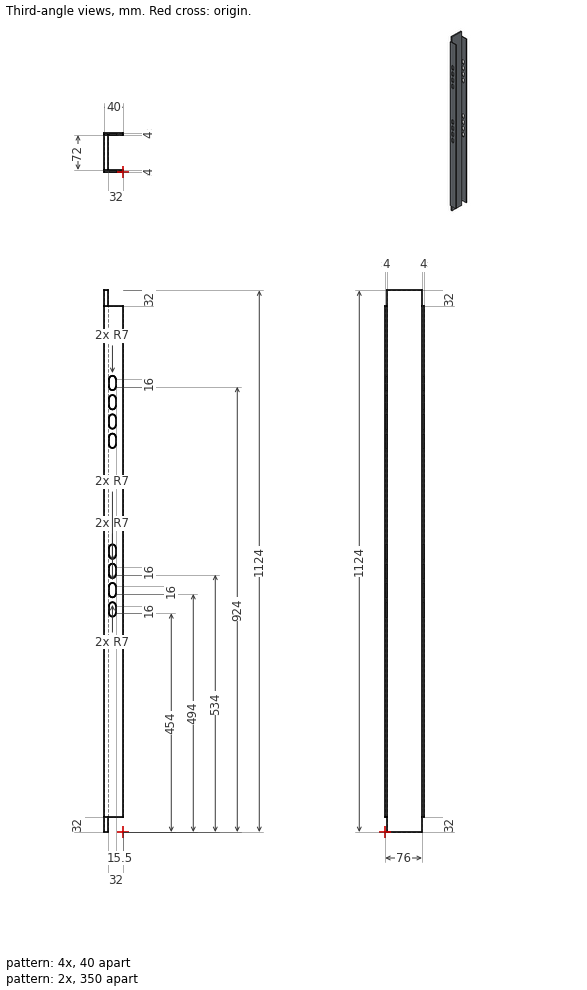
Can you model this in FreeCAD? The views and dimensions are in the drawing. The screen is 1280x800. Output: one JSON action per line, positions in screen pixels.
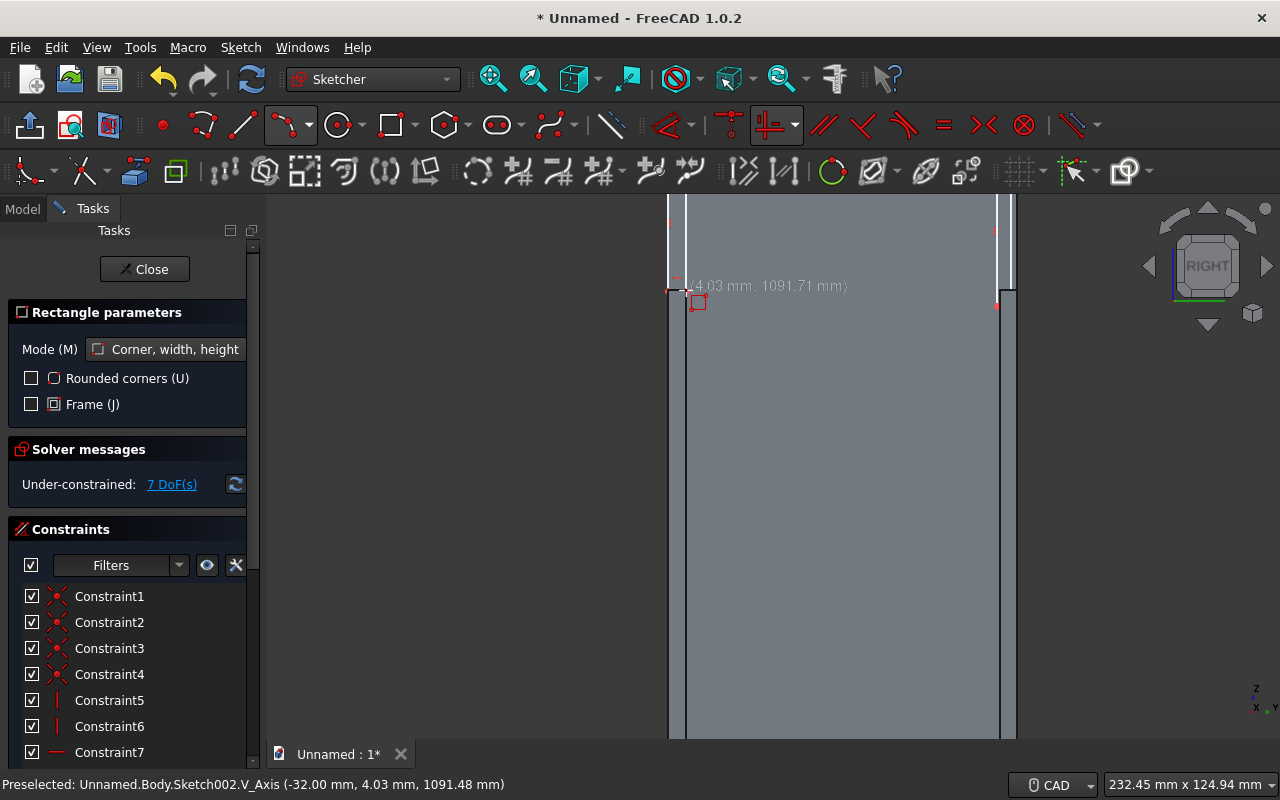
{"action": "scroll", "coordinate": [693, 295], "scroll_direction": "down", "scroll_amount": 13}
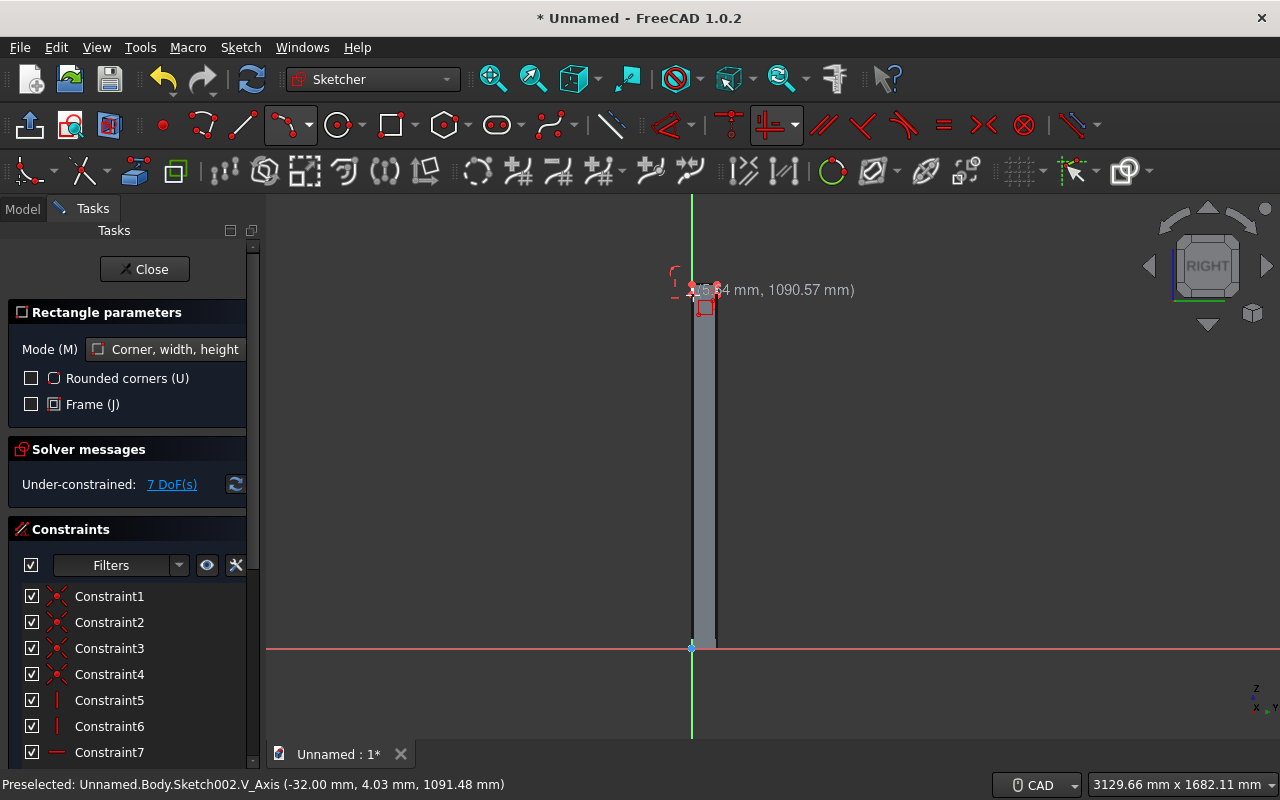
{"action": "scroll", "coordinate": [716, 638], "scroll_direction": "up", "scroll_amount": 13}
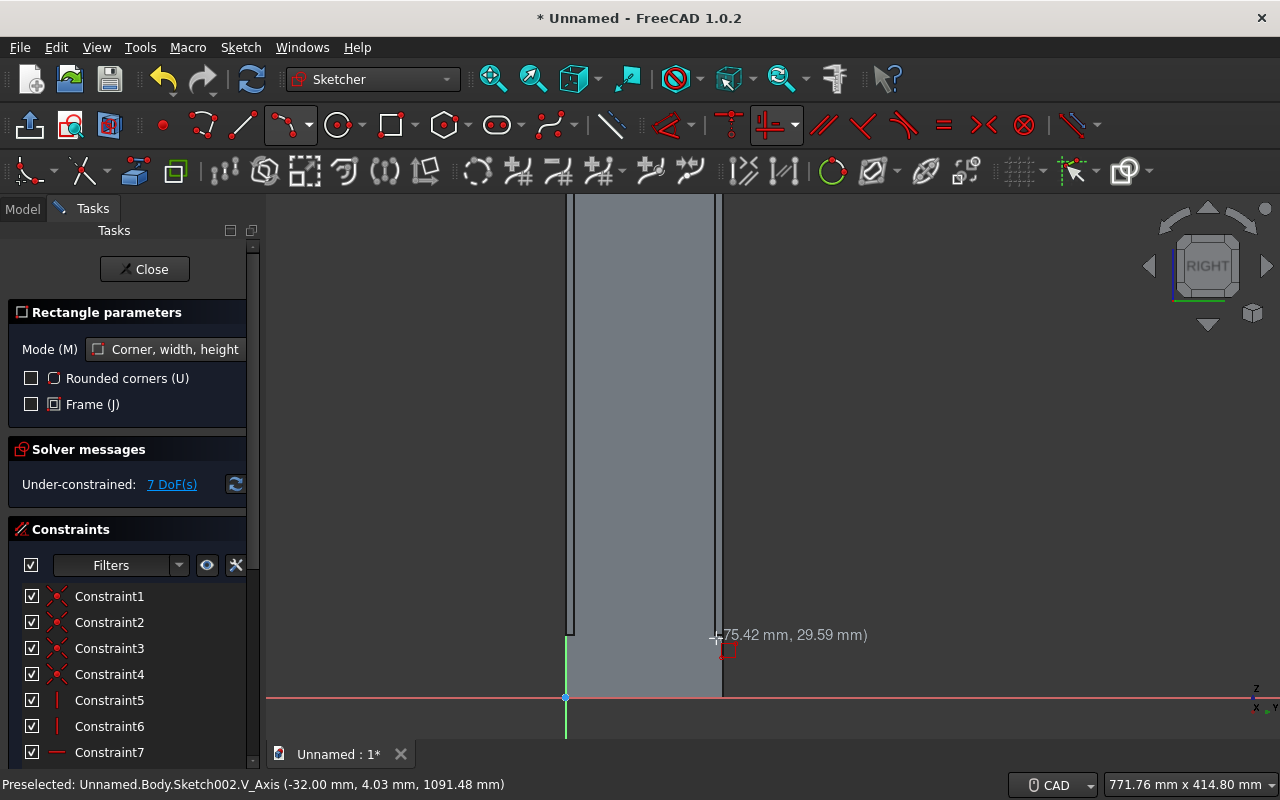
{"action": "scroll", "coordinate": [716, 639], "scroll_direction": "down", "scroll_amount": 13}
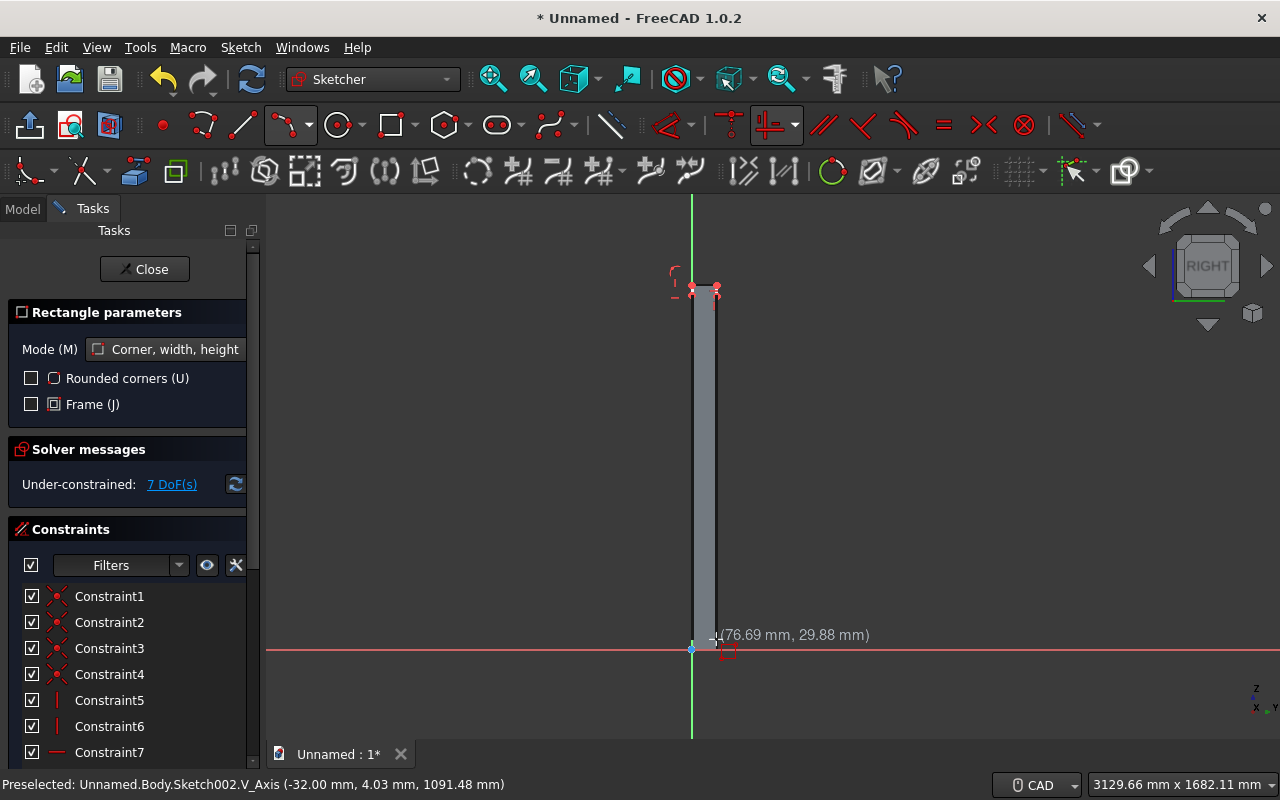
{"action": "scroll", "coordinate": [716, 639], "scroll_direction": "up", "scroll_amount": 3}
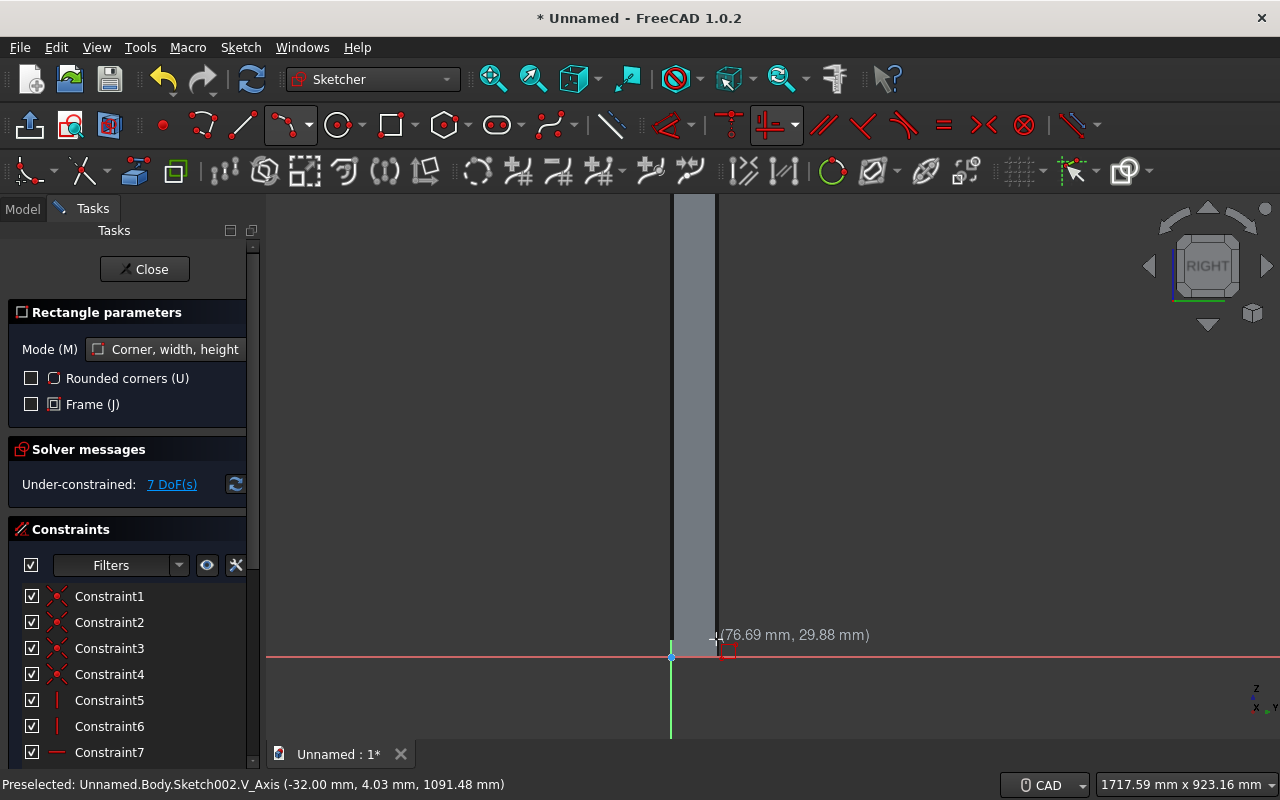
{"action": "left_click", "coordinate": [716, 639]}
{"action": "left_click", "coordinate": [718, 657]}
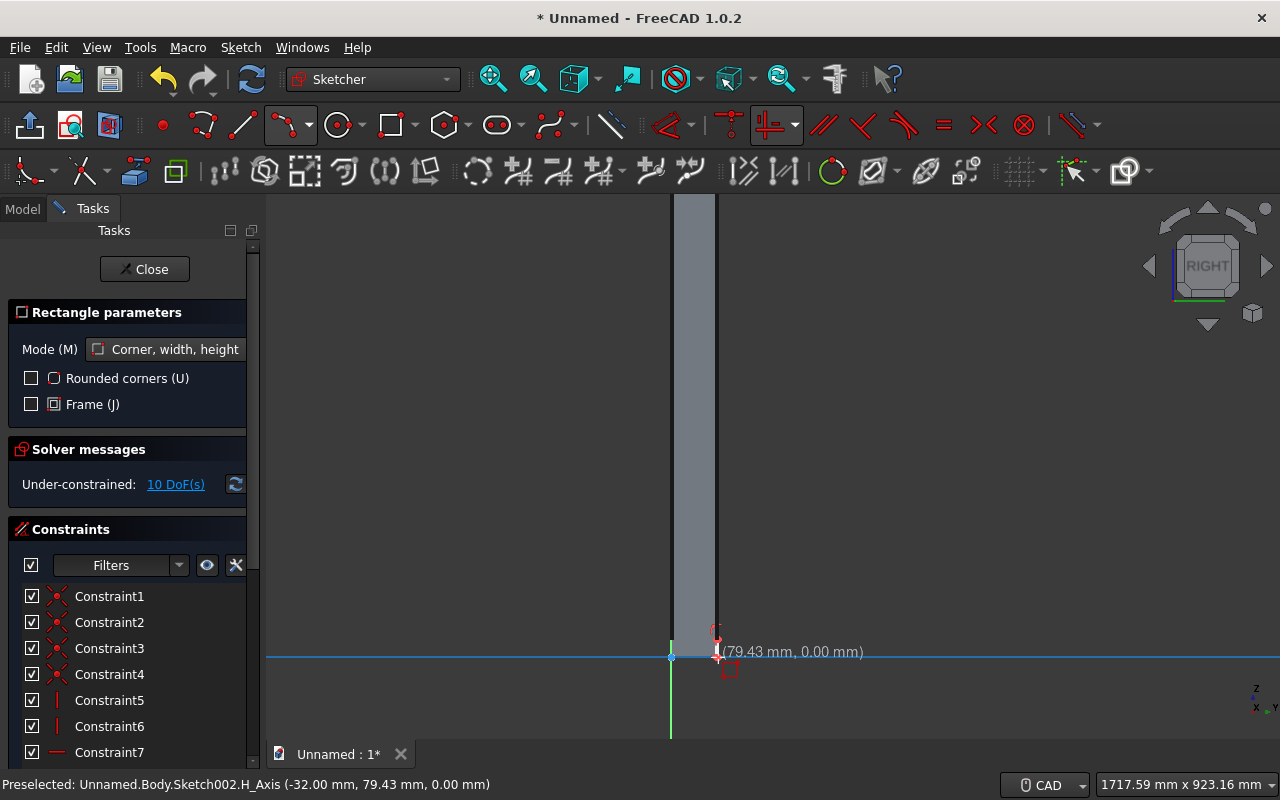
{"action": "scroll", "coordinate": [671, 657], "scroll_direction": "up", "scroll_amount": 10}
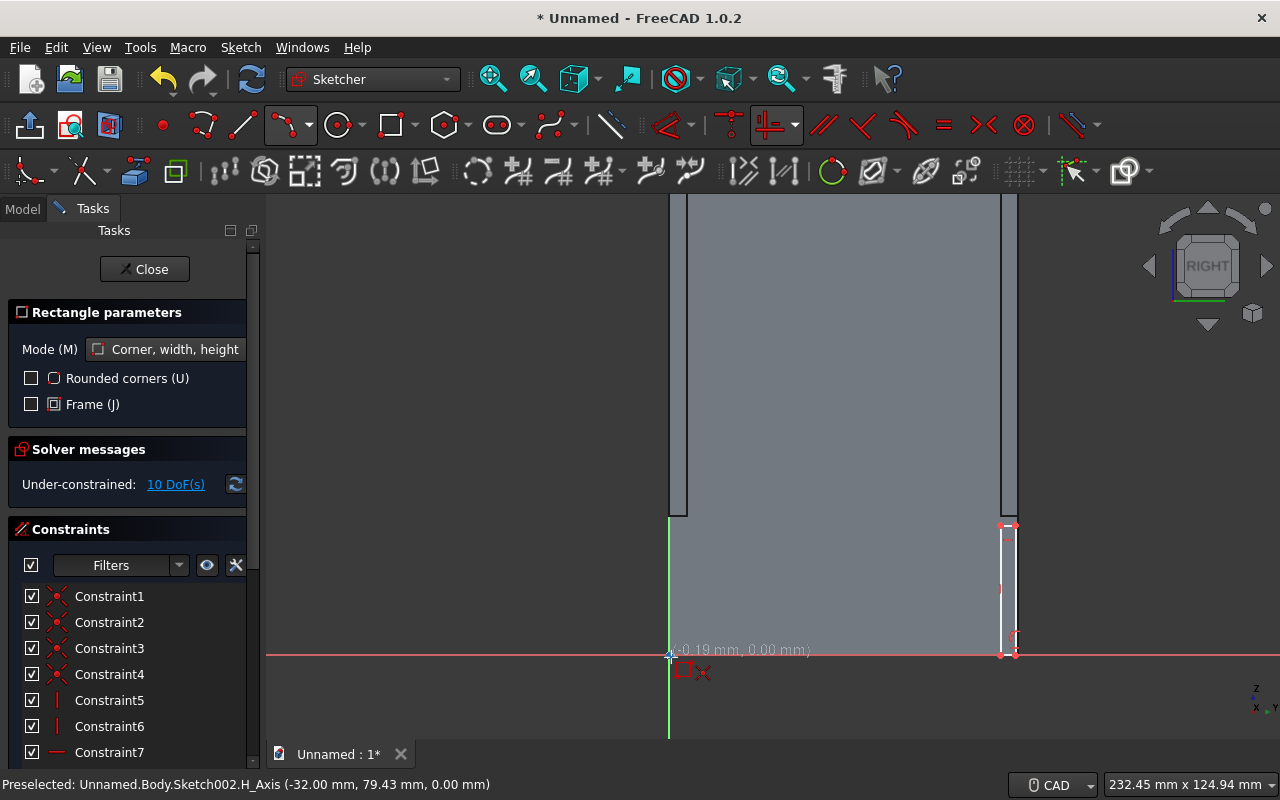
{"action": "scroll", "coordinate": [693, 648], "scroll_direction": "down", "scroll_amount": 13}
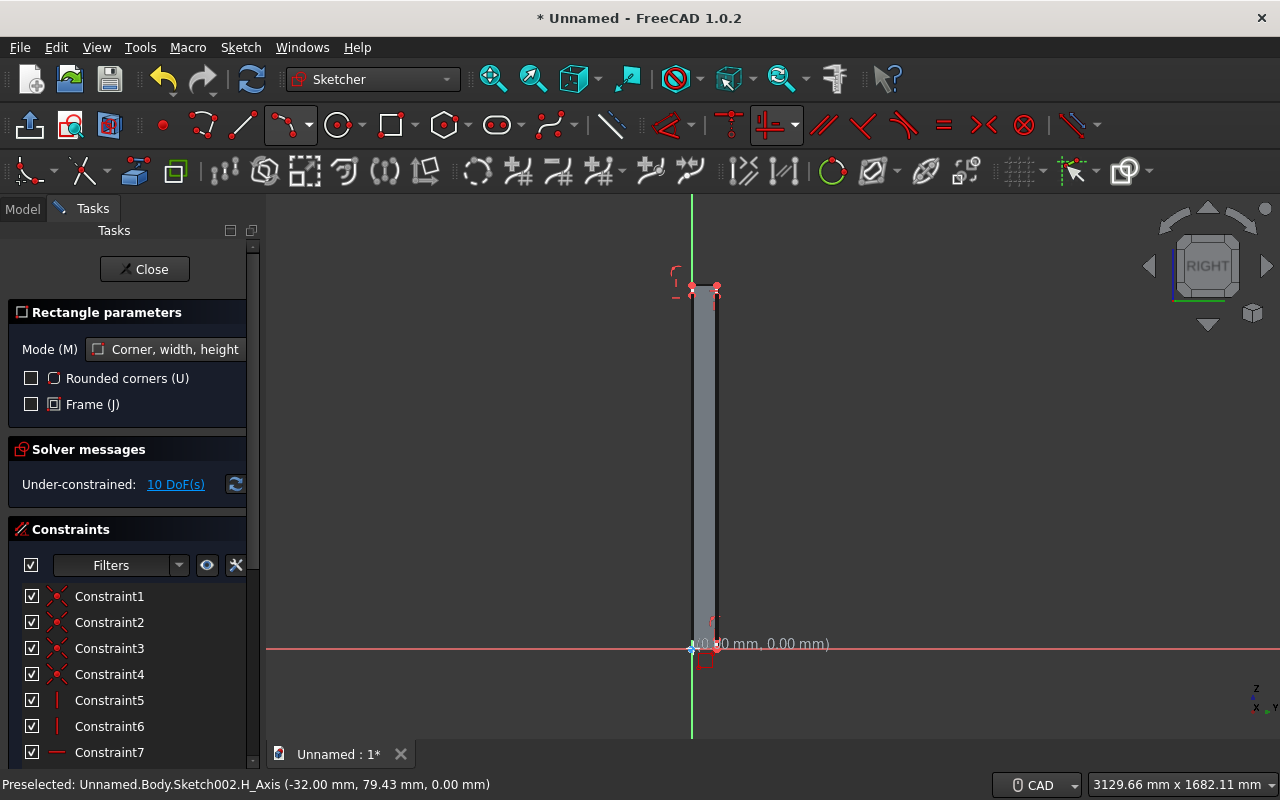
{"action": "left_click", "coordinate": [692, 649]}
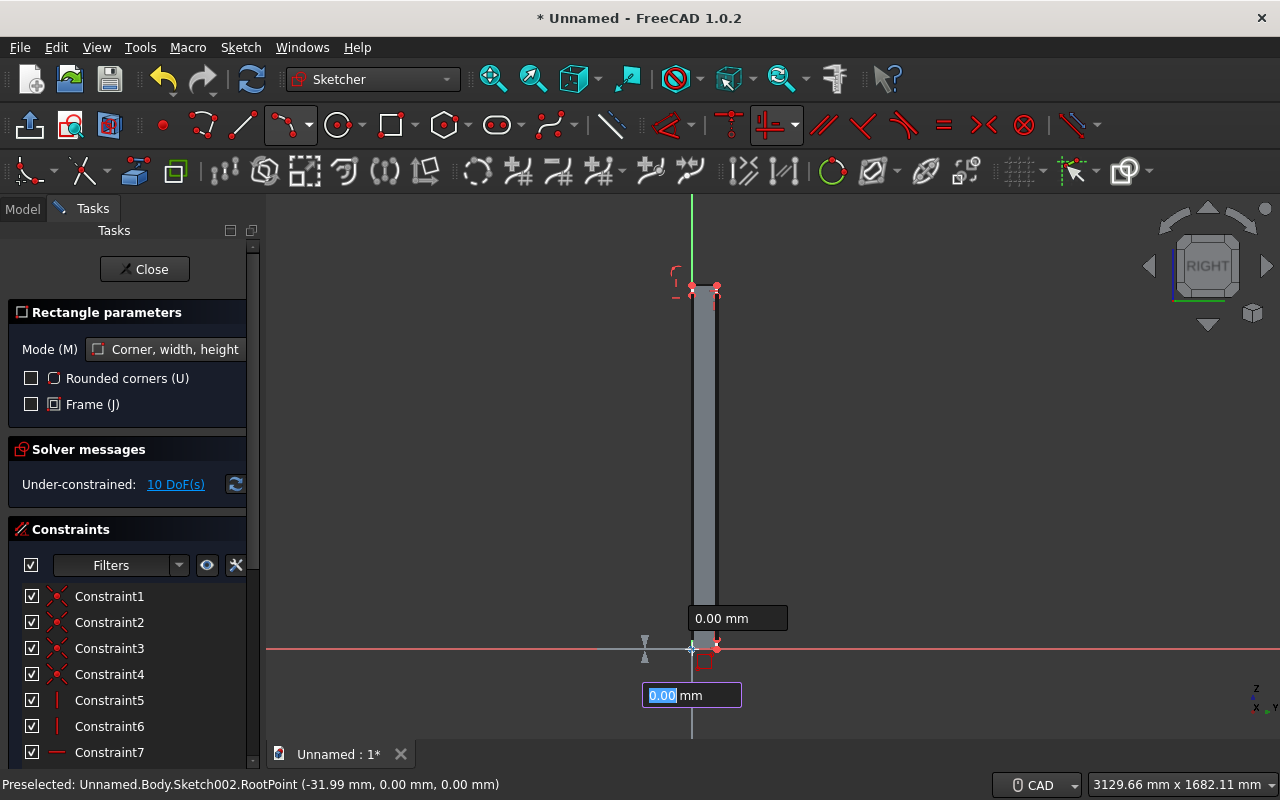
{"action": "scroll", "coordinate": [693, 639], "scroll_direction": "up", "scroll_amount": 13}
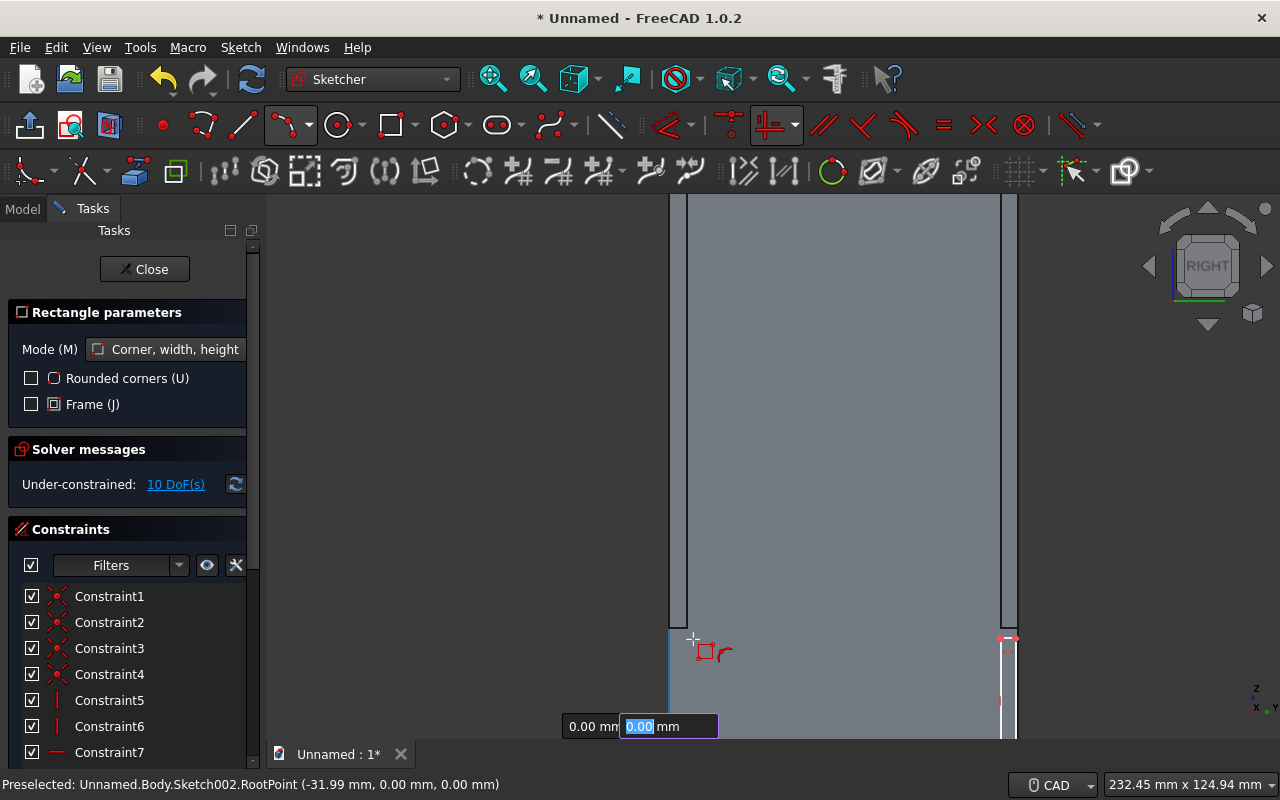
{"action": "left_click", "coordinate": [687, 628]}
{"action": "key", "text": "Escape"}